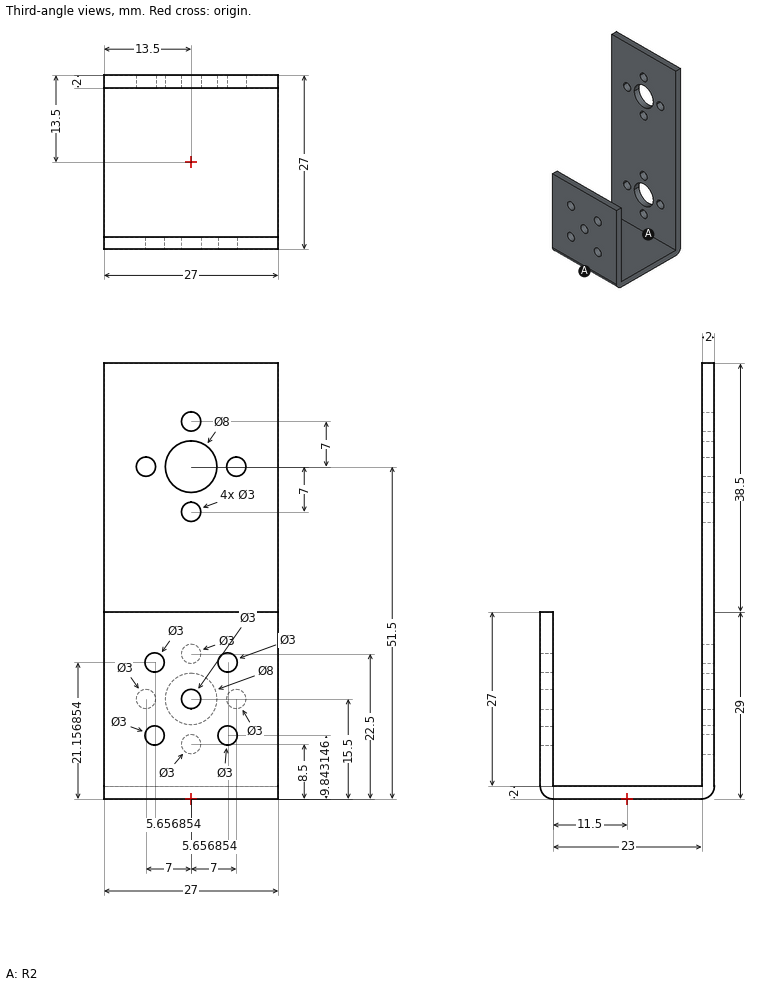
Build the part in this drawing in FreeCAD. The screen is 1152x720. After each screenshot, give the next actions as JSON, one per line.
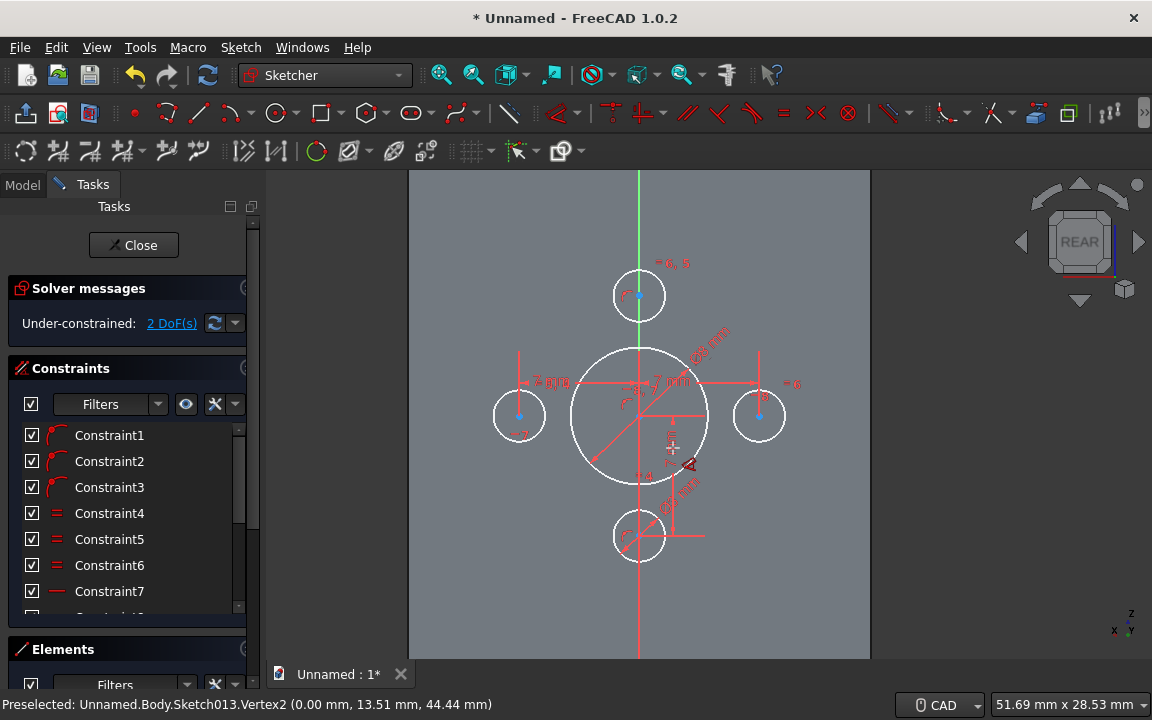
{"action": "left_click", "coordinate": [639, 416]}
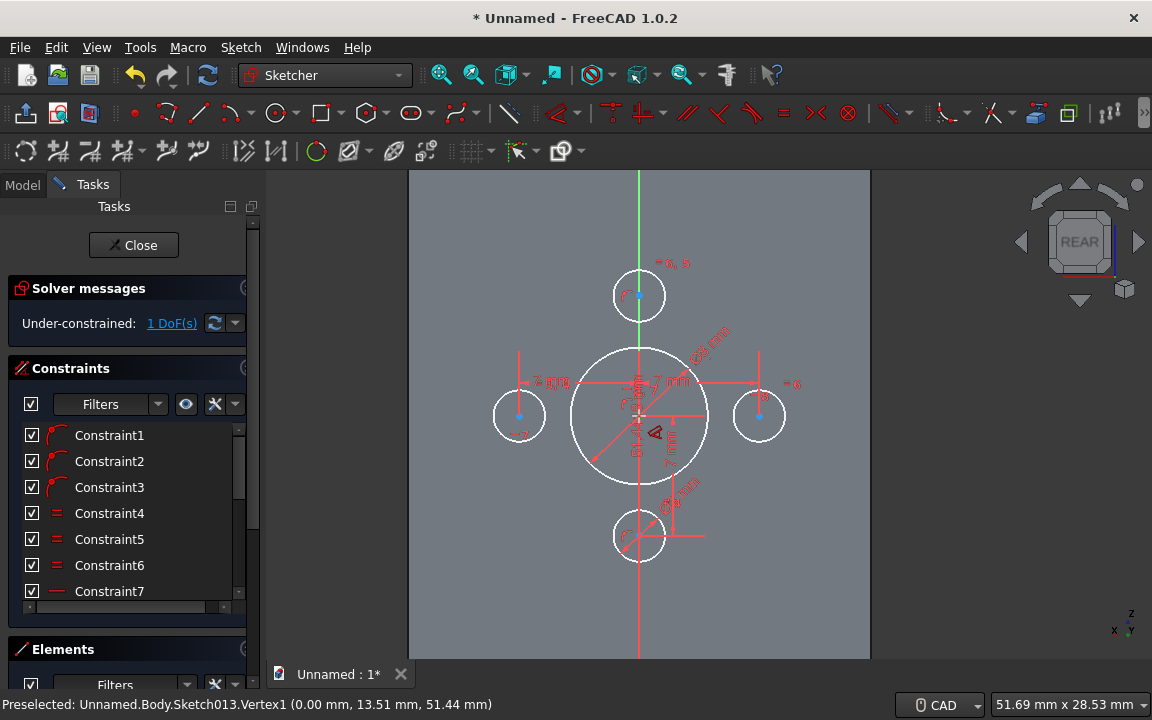
{"action": "left_click", "coordinate": [639, 296]}
{"action": "left_click", "coordinate": [605, 328]}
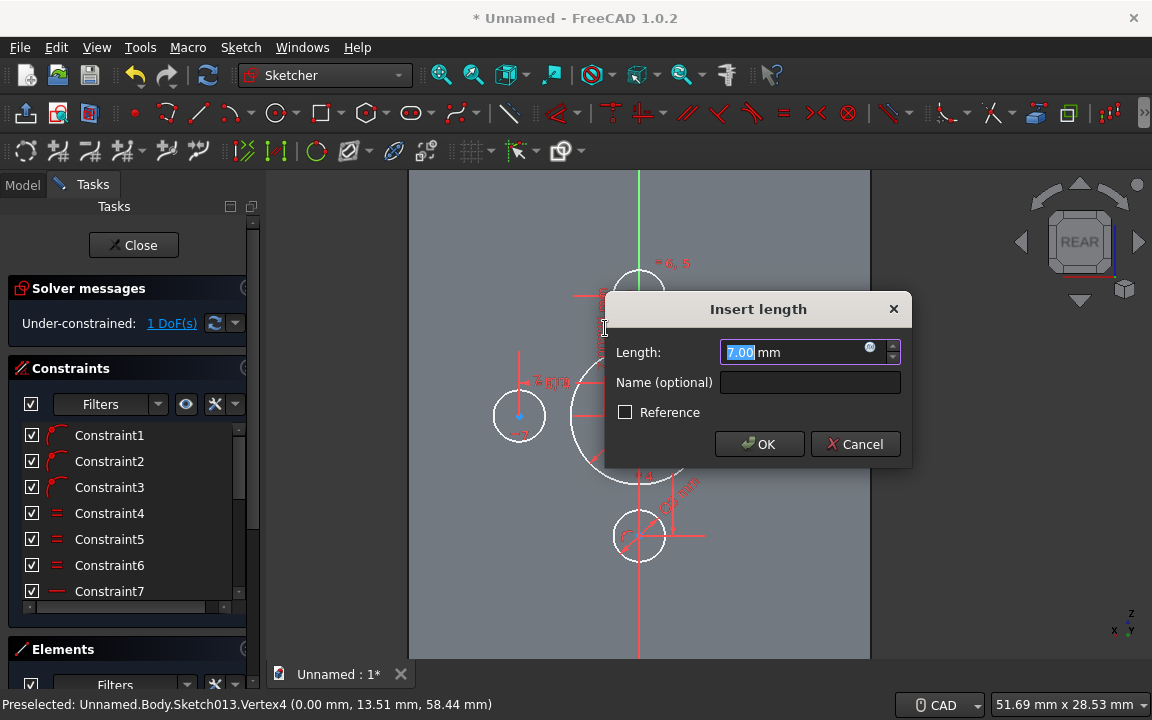
{"action": "type", "text": "7"}
{"action": "key", "text": "Return"}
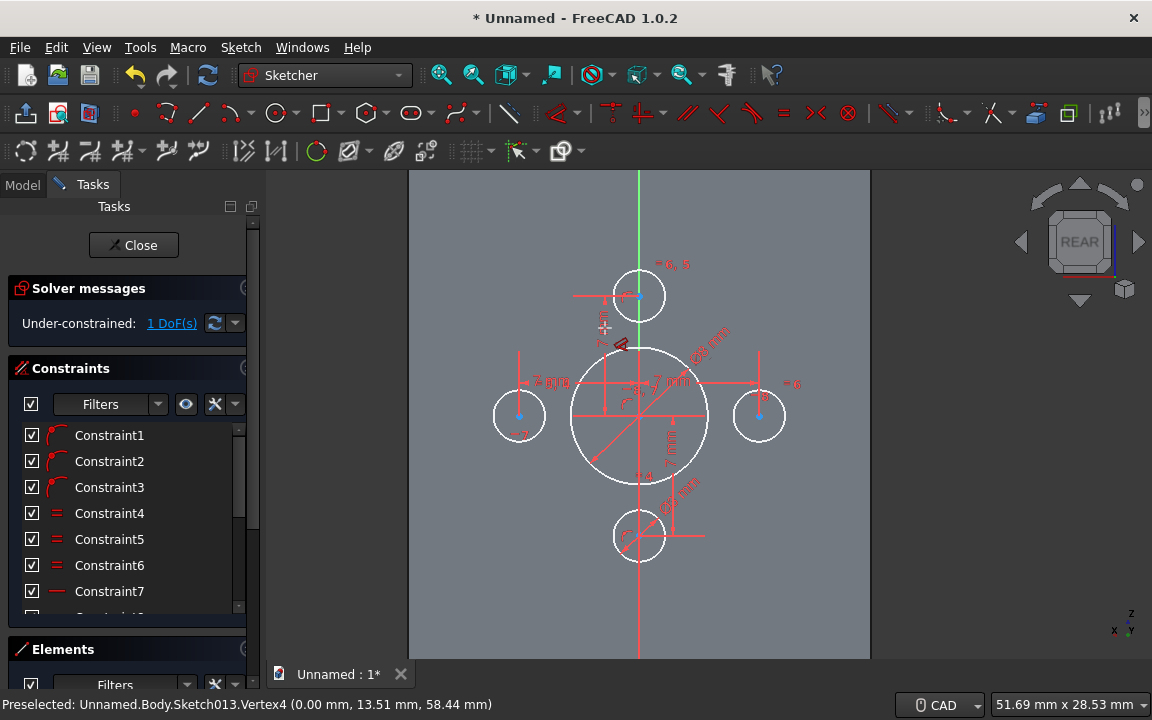
{"action": "left_click", "coordinate": [639, 416]}
{"action": "left_click", "coordinate": [673, 573]}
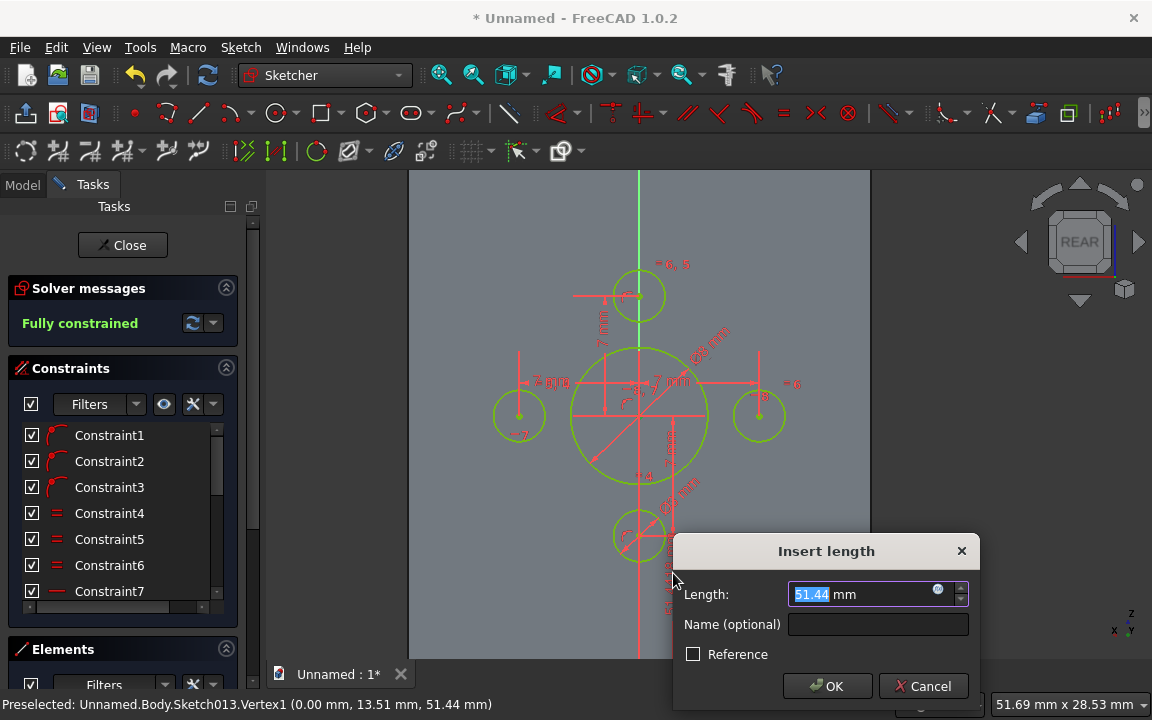
{"action": "type", "text": "51.5"}
{"action": "key", "text": "Return"}
{"action": "key", "text": "Escape"}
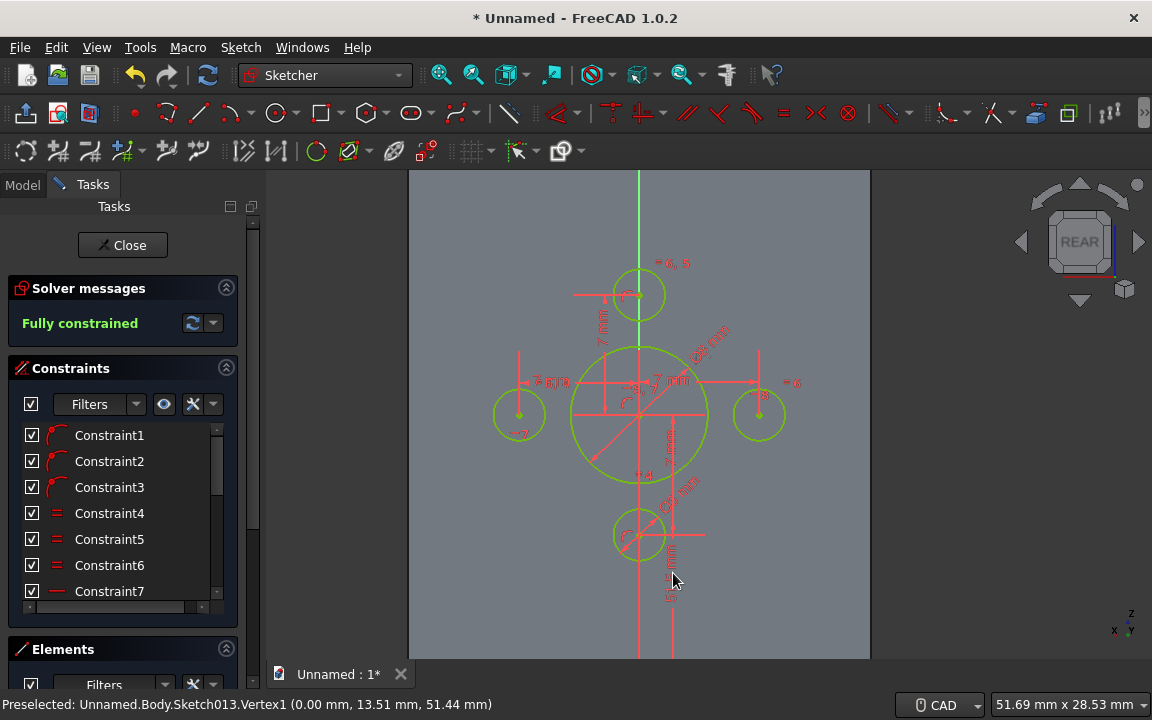
{"action": "left_click", "coordinate": [123, 245]}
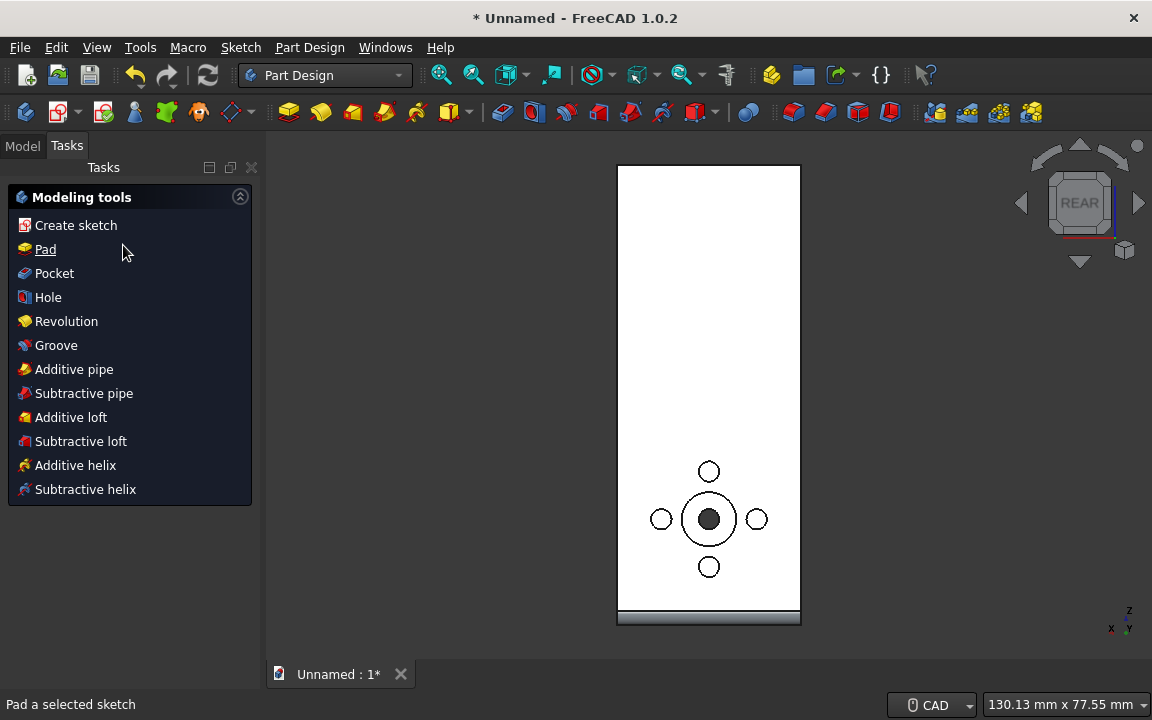
{"action": "left_click", "coordinate": [504, 112]}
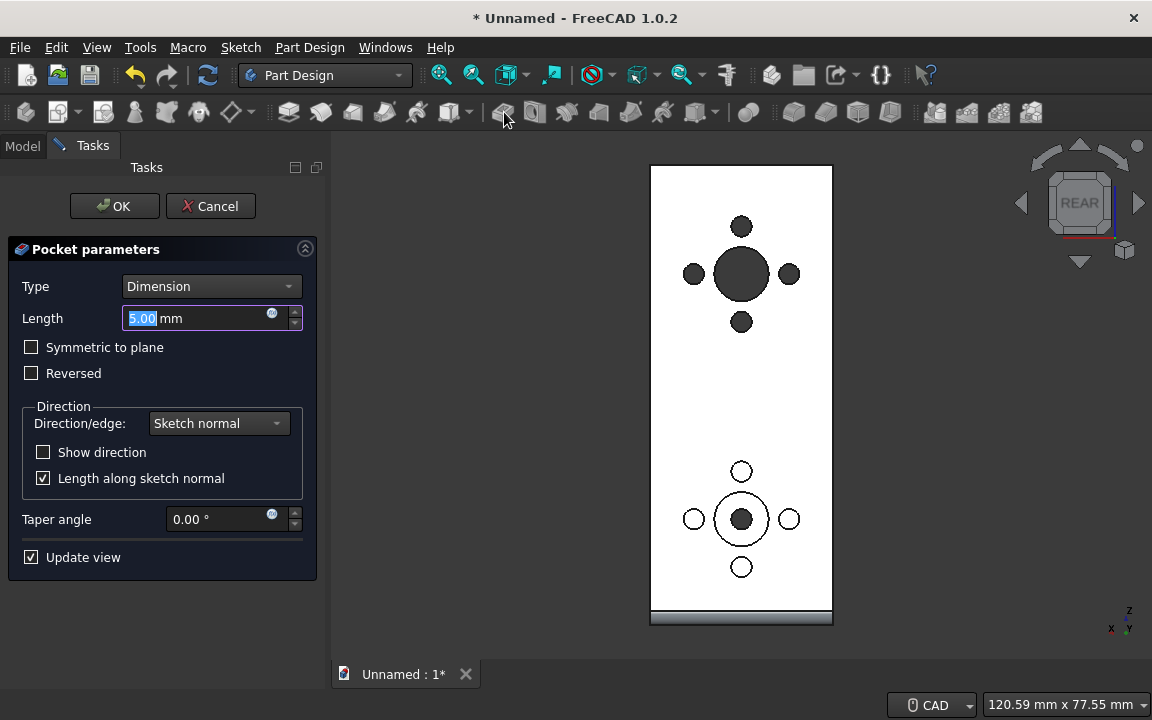
{"action": "type", "text": "2"}
{"action": "key", "text": "Tab"}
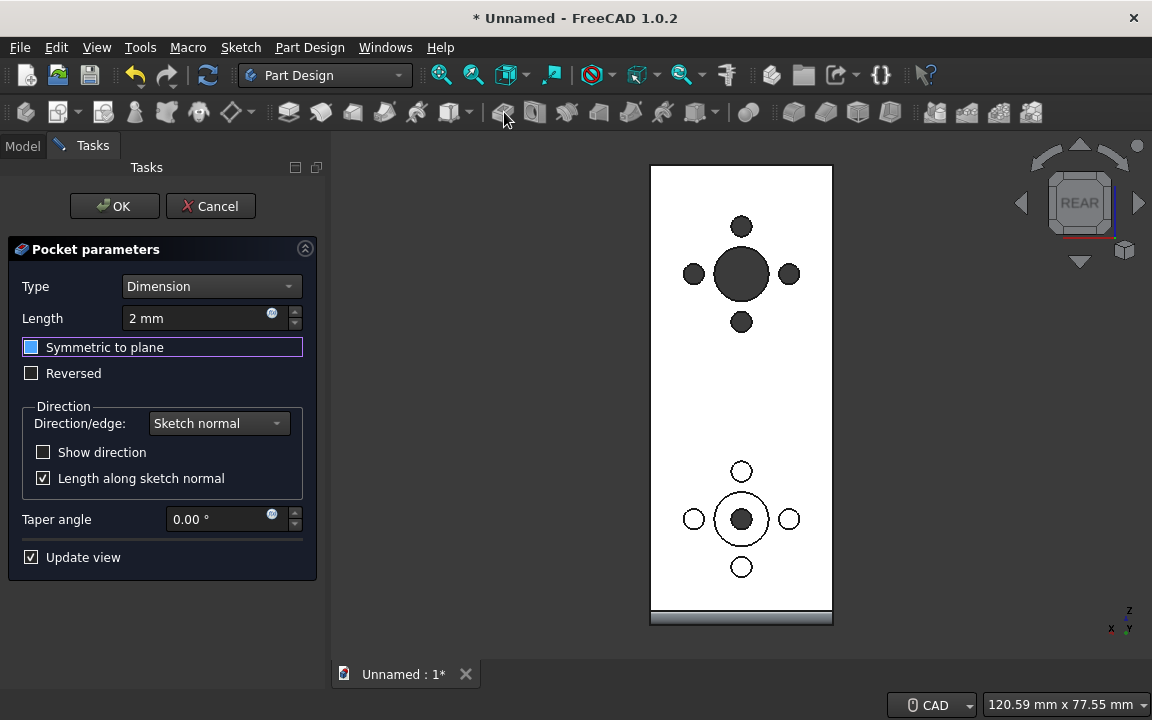
{"action": "left_click", "coordinate": [115, 206]}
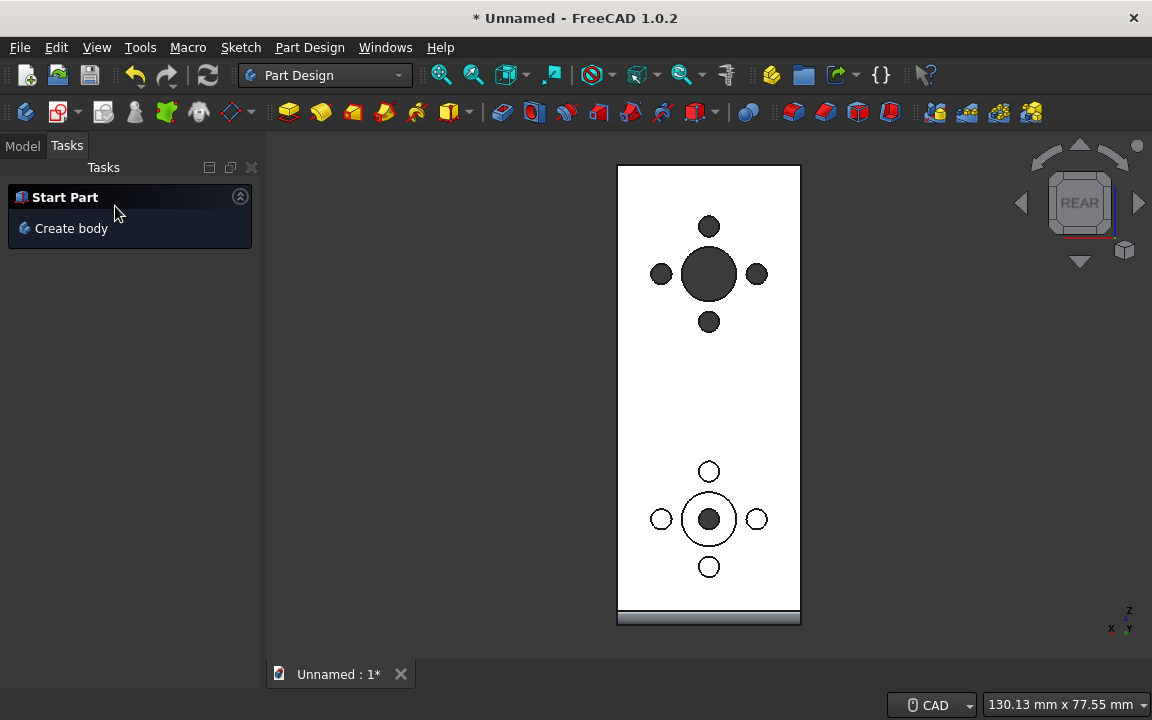
{"action": "key", "text": "0"}